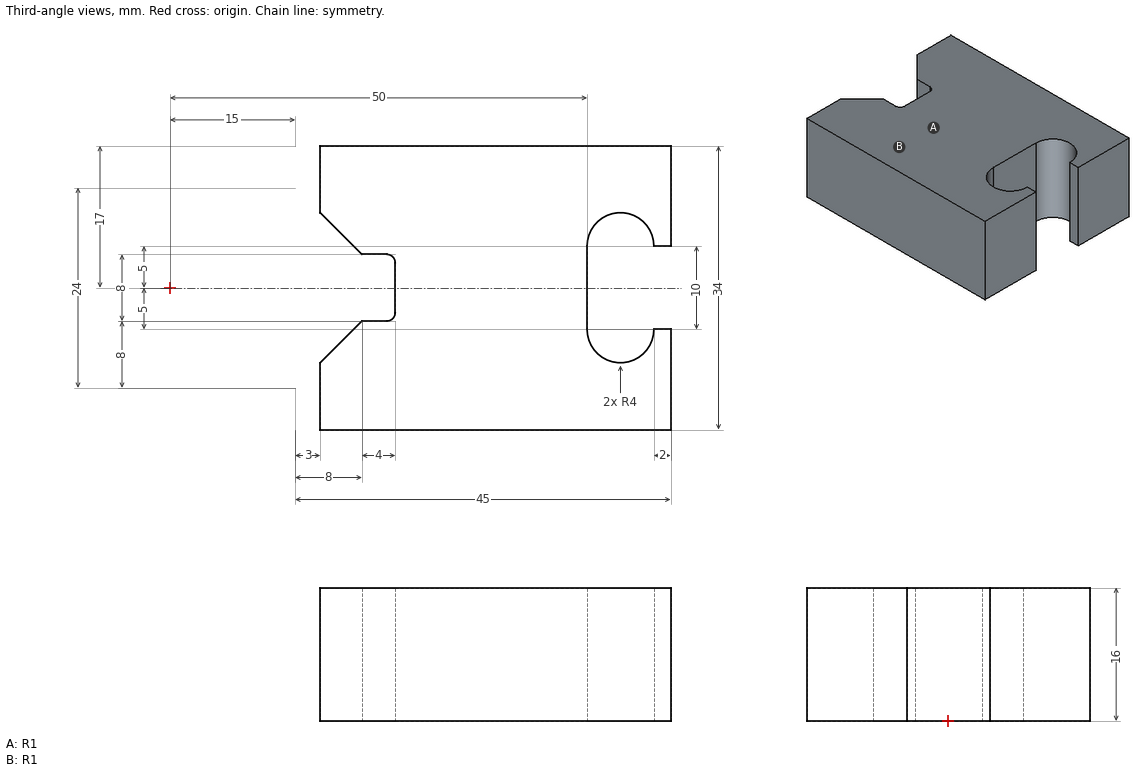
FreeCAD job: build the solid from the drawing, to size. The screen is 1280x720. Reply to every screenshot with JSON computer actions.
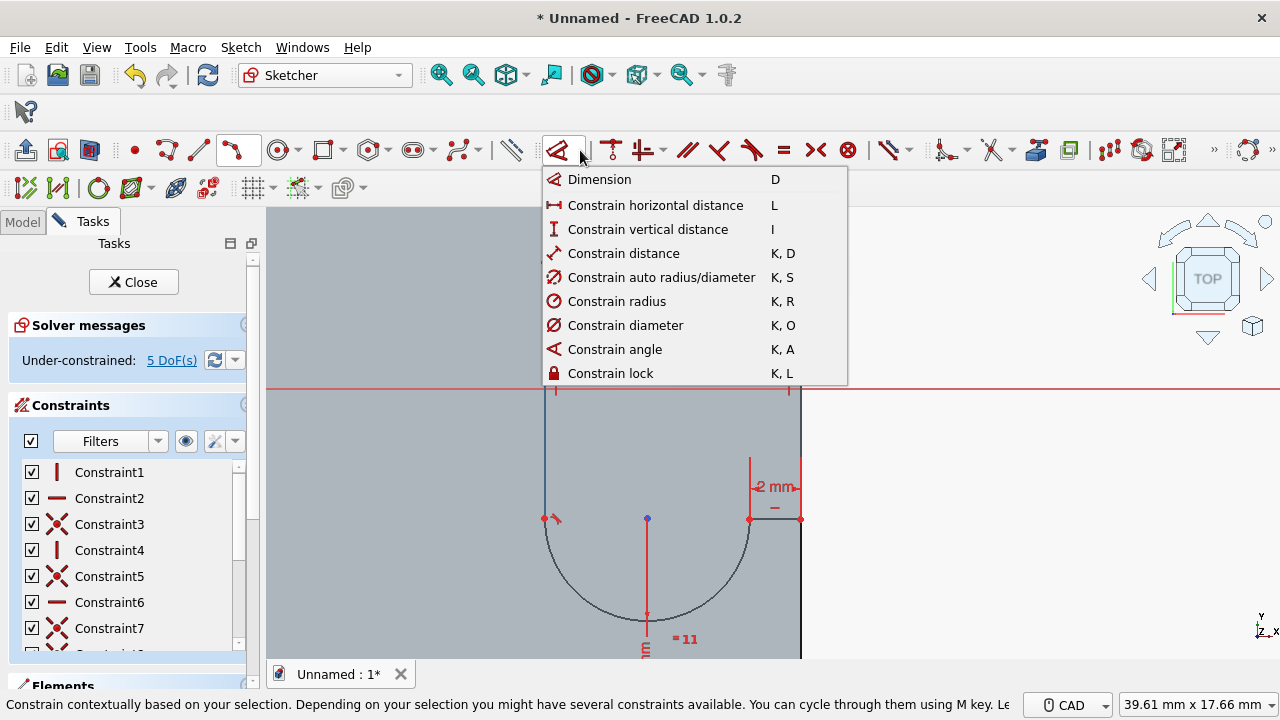
{"action": "left_click", "coordinate": [695, 229]}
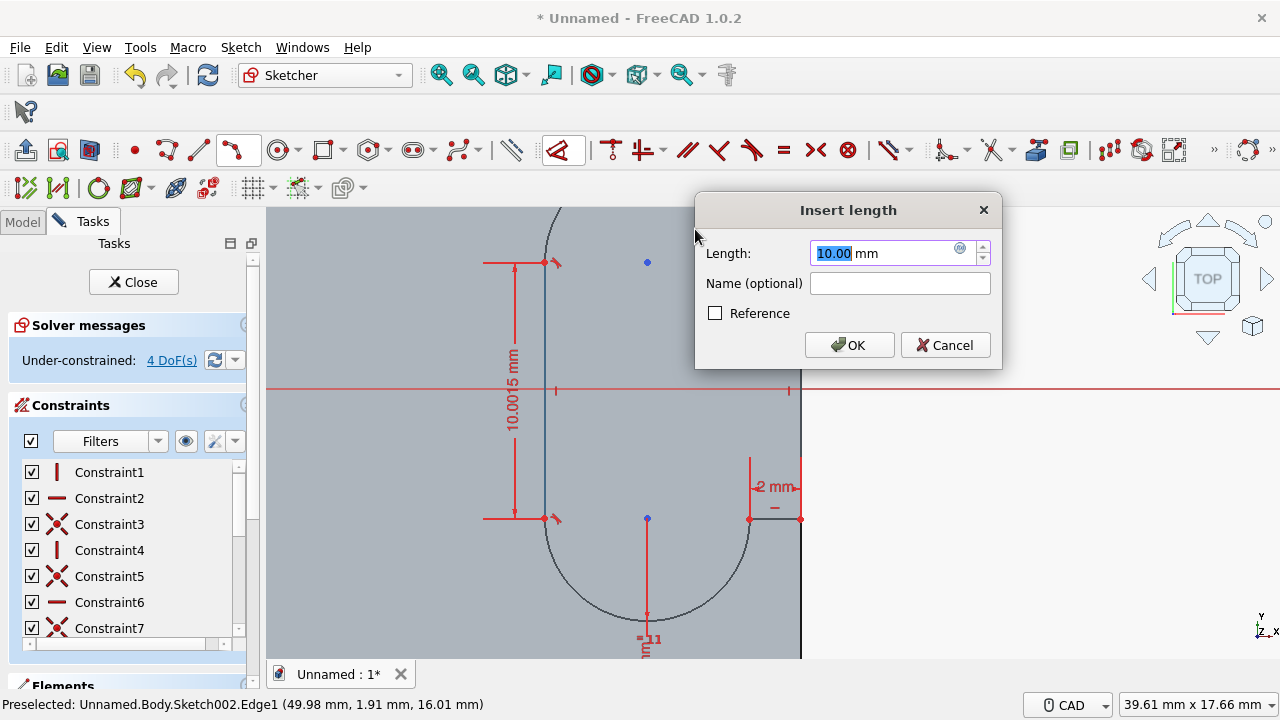
{"action": "type", "text": "10"}
{"action": "key", "text": "Return"}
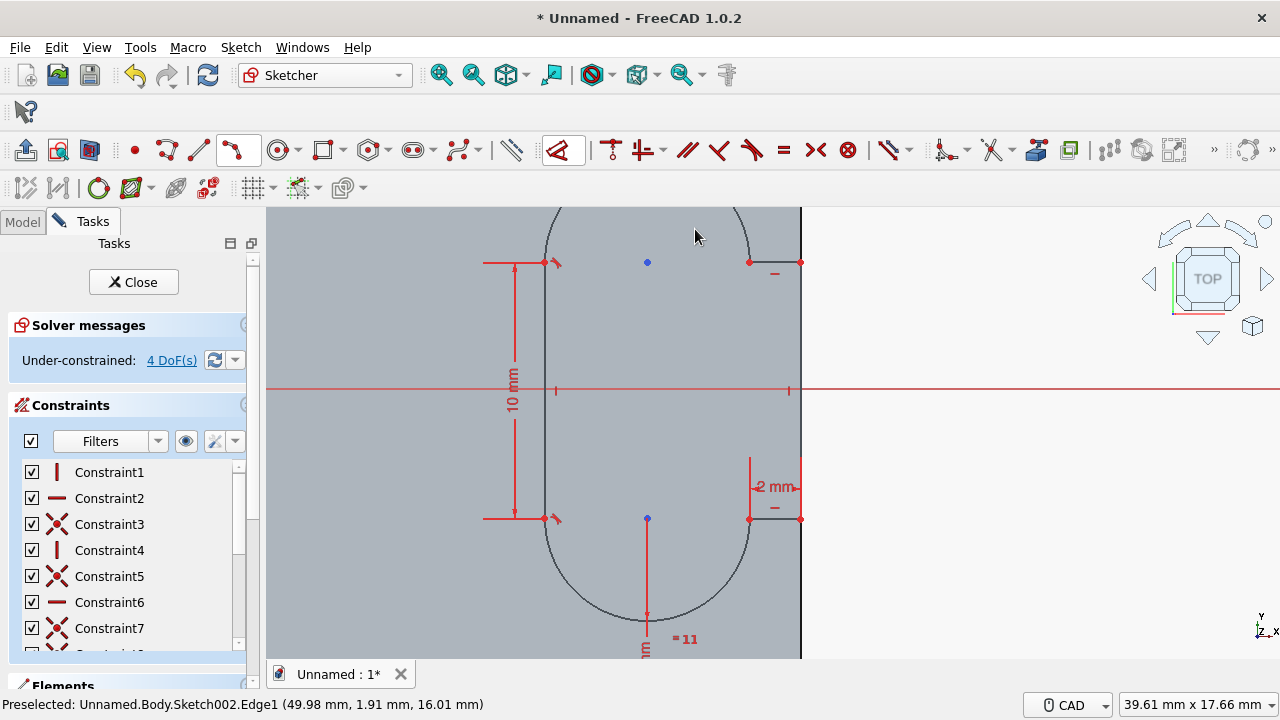
{"action": "left_click", "coordinate": [801, 442]}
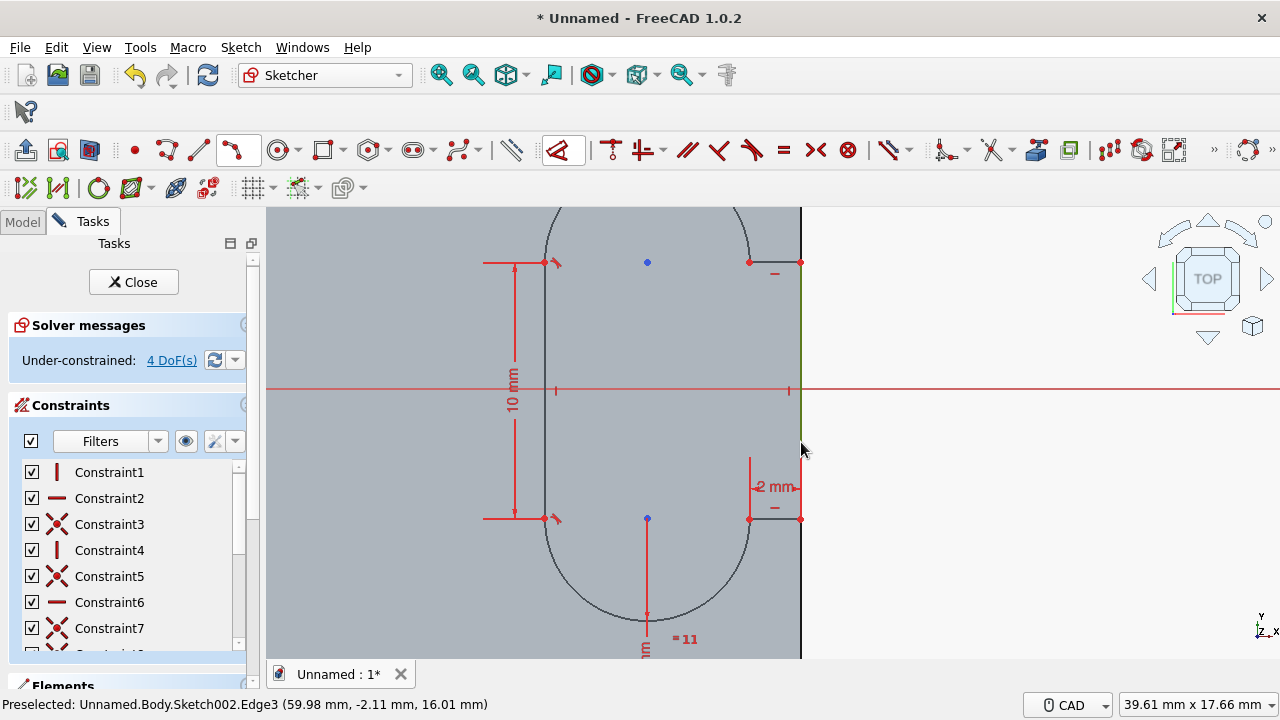
{"action": "left_click", "coordinate": [580, 150]}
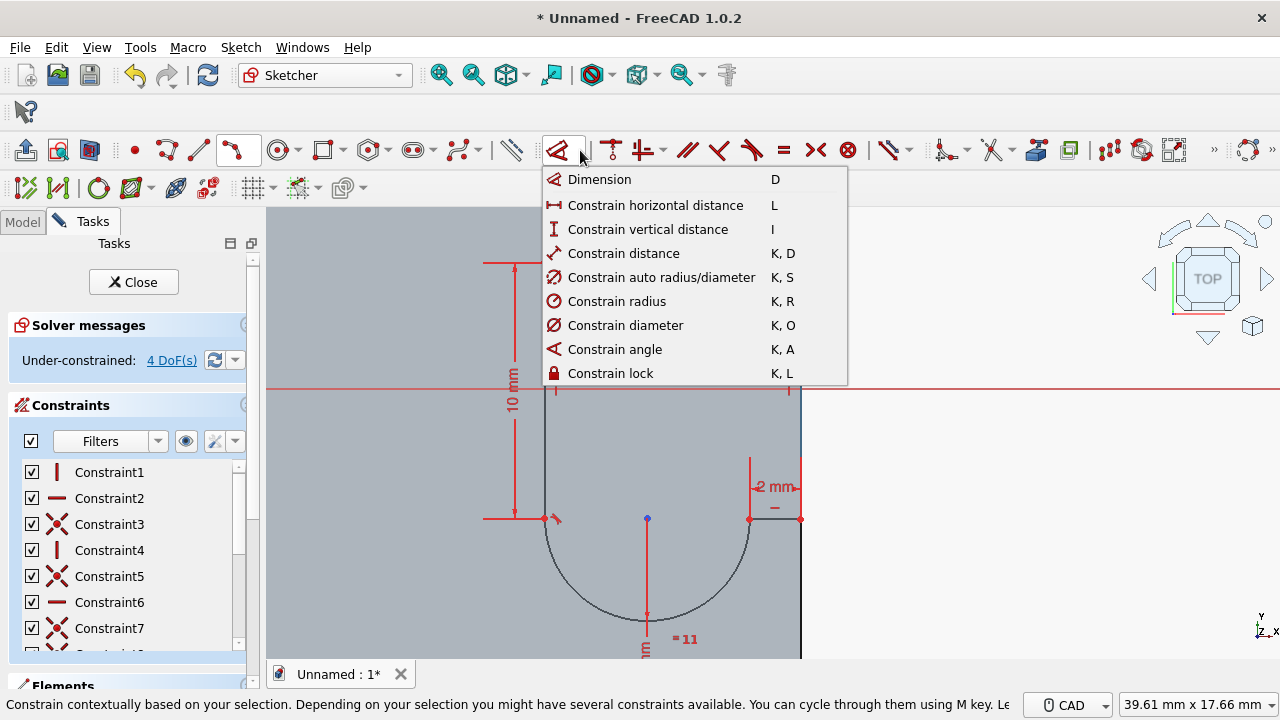
{"action": "left_click", "coordinate": [695, 229]}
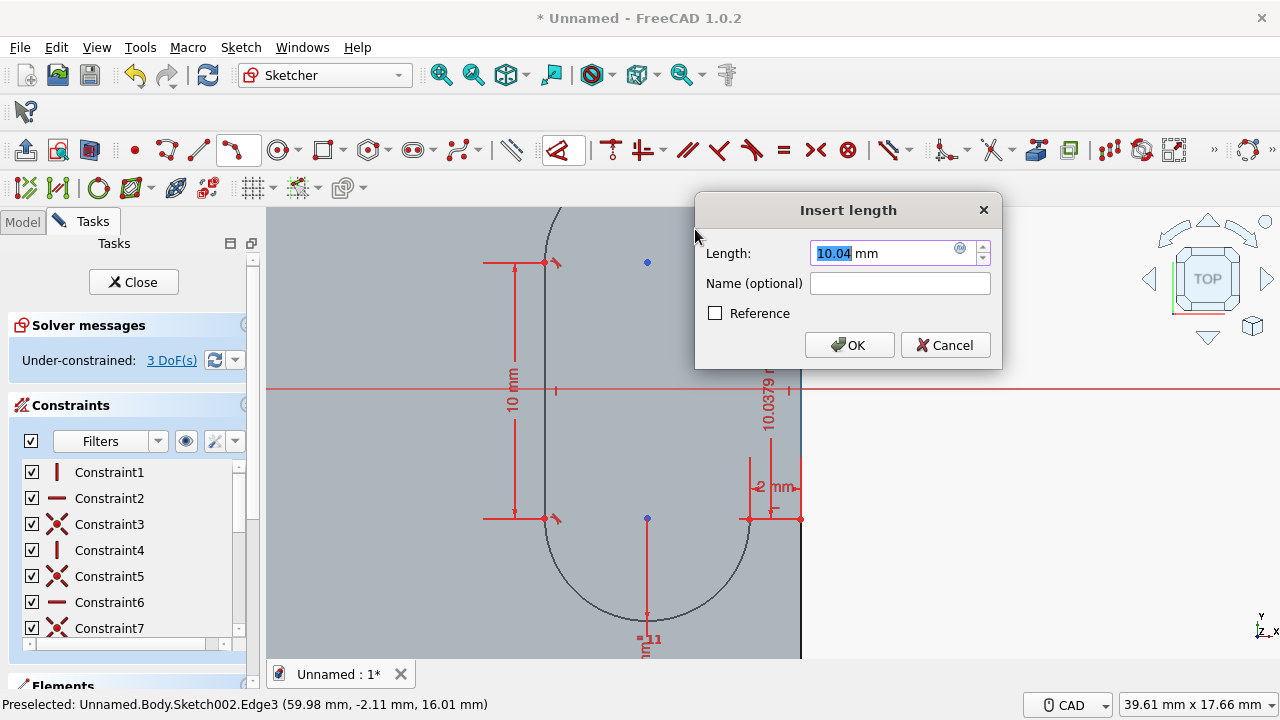
{"action": "type", "text": "10"}
{"action": "key", "text": "Return"}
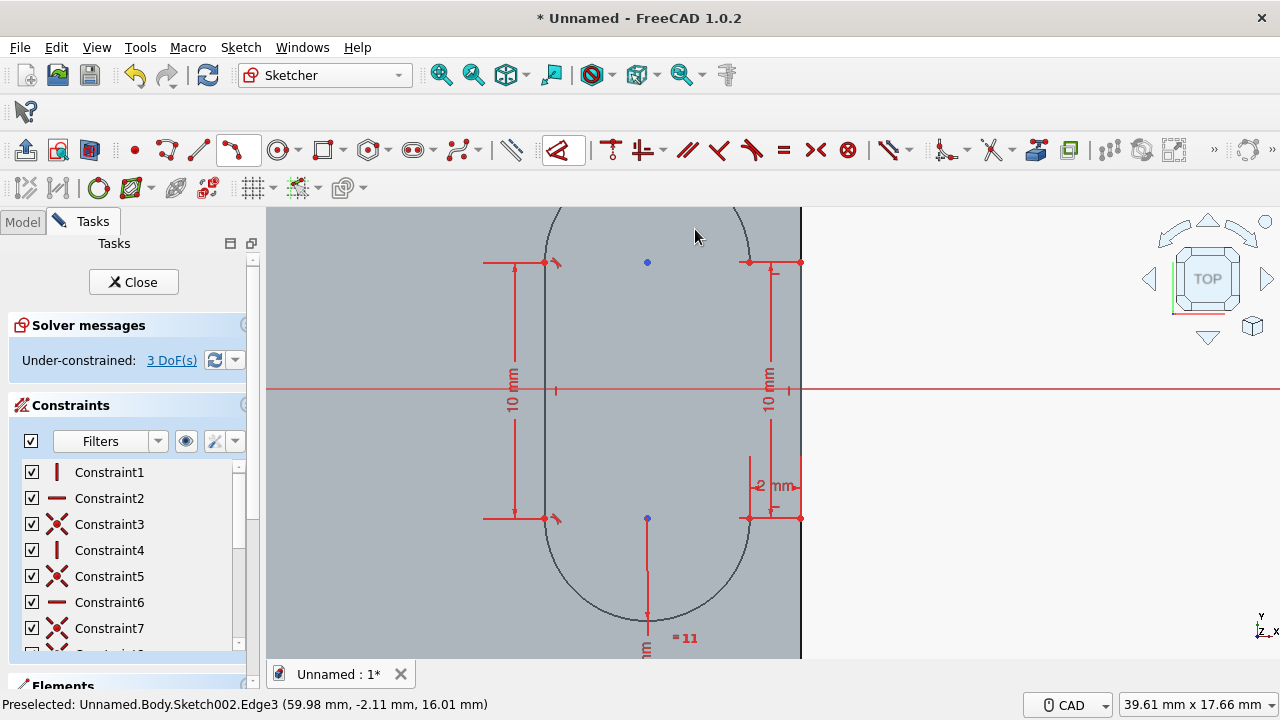
{"action": "left_click", "coordinate": [545, 263]}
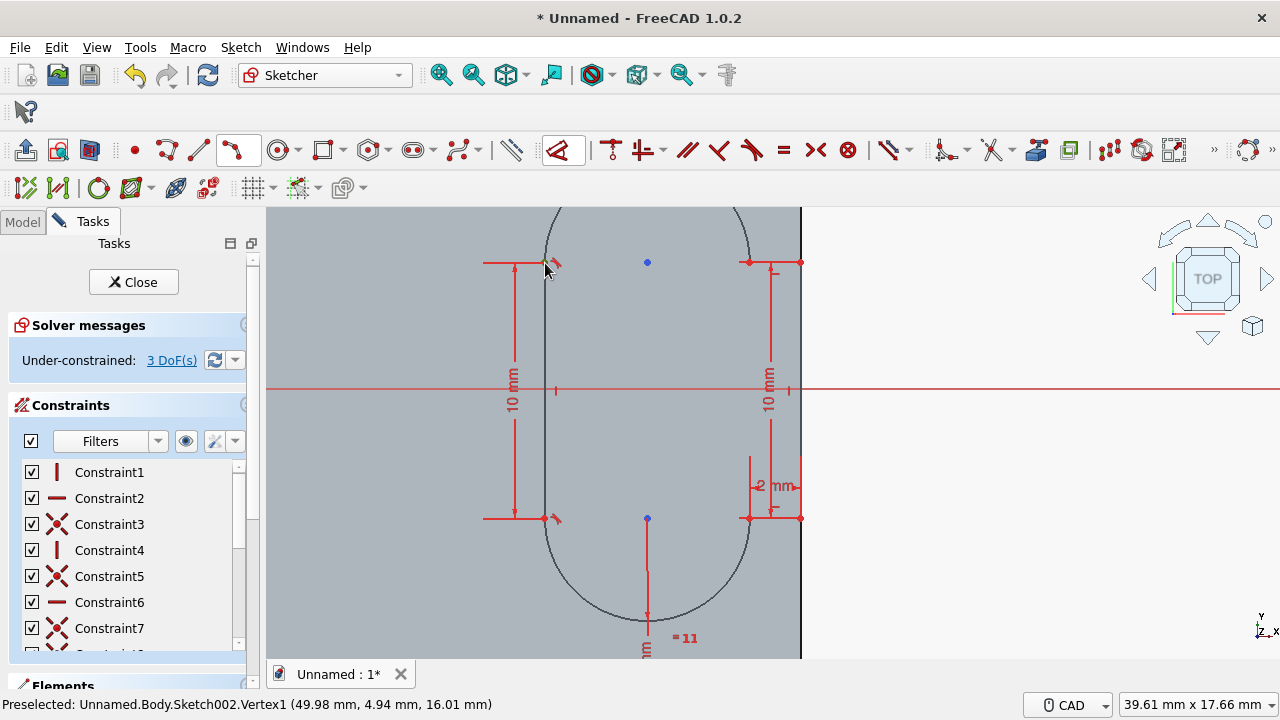
{"action": "key", "text": "i"}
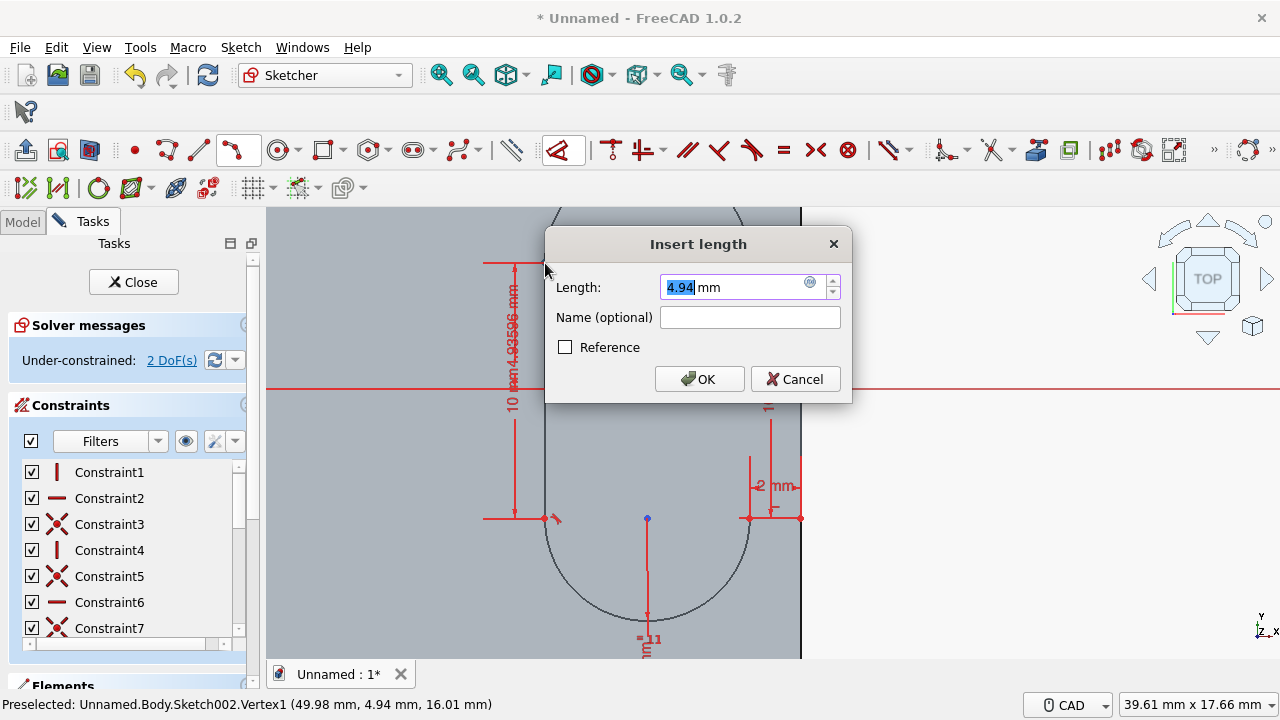
{"action": "type", "text": "5"}
{"action": "key", "text": "Return"}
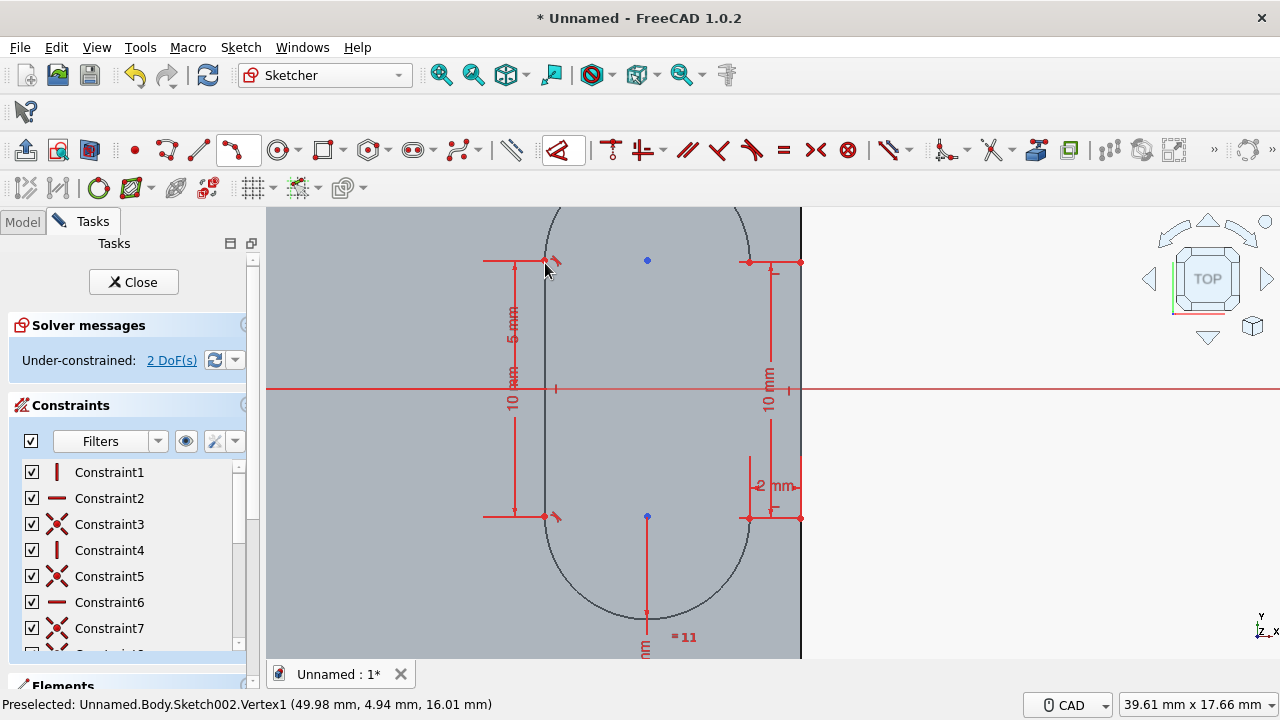
{"action": "left_click", "coordinate": [750, 518]}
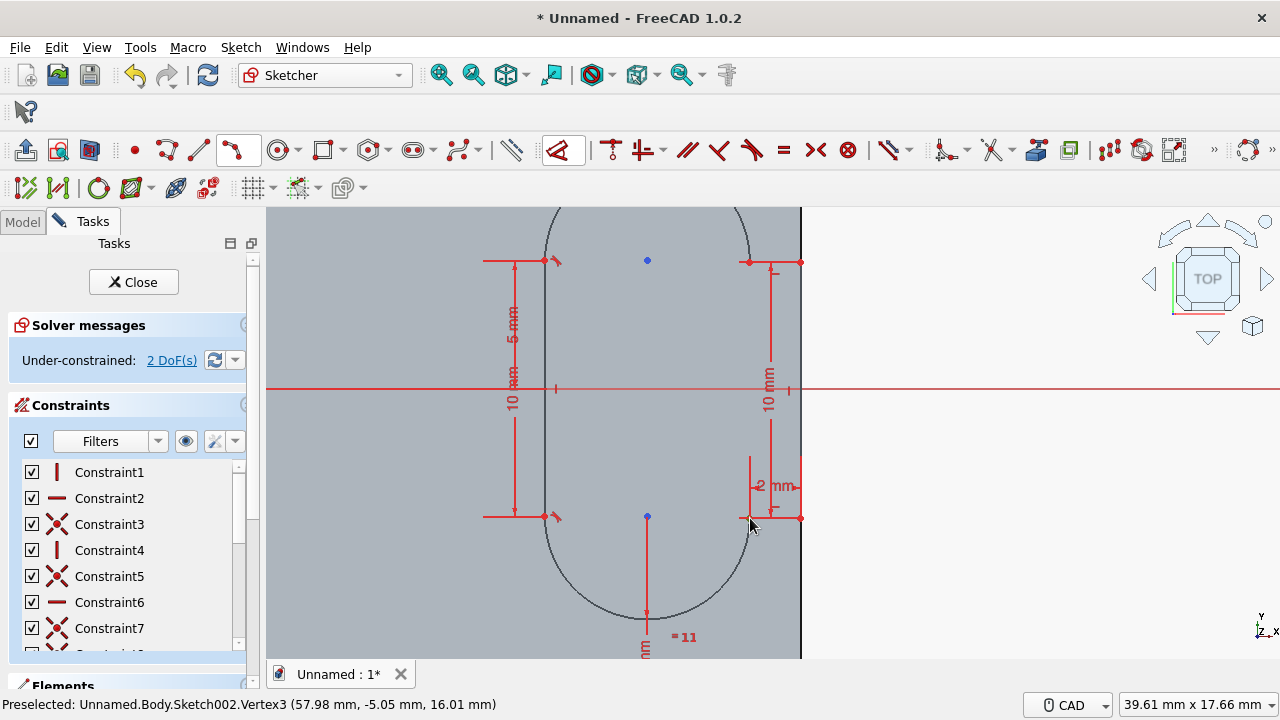
{"action": "left_click", "coordinate": [580, 150]}